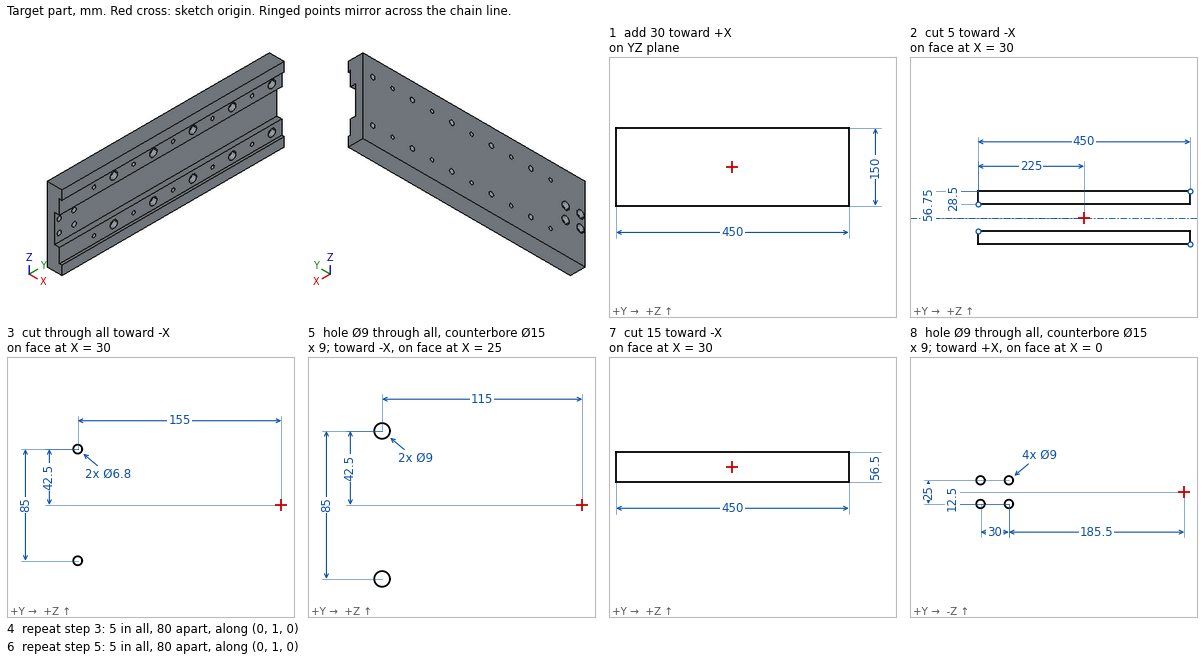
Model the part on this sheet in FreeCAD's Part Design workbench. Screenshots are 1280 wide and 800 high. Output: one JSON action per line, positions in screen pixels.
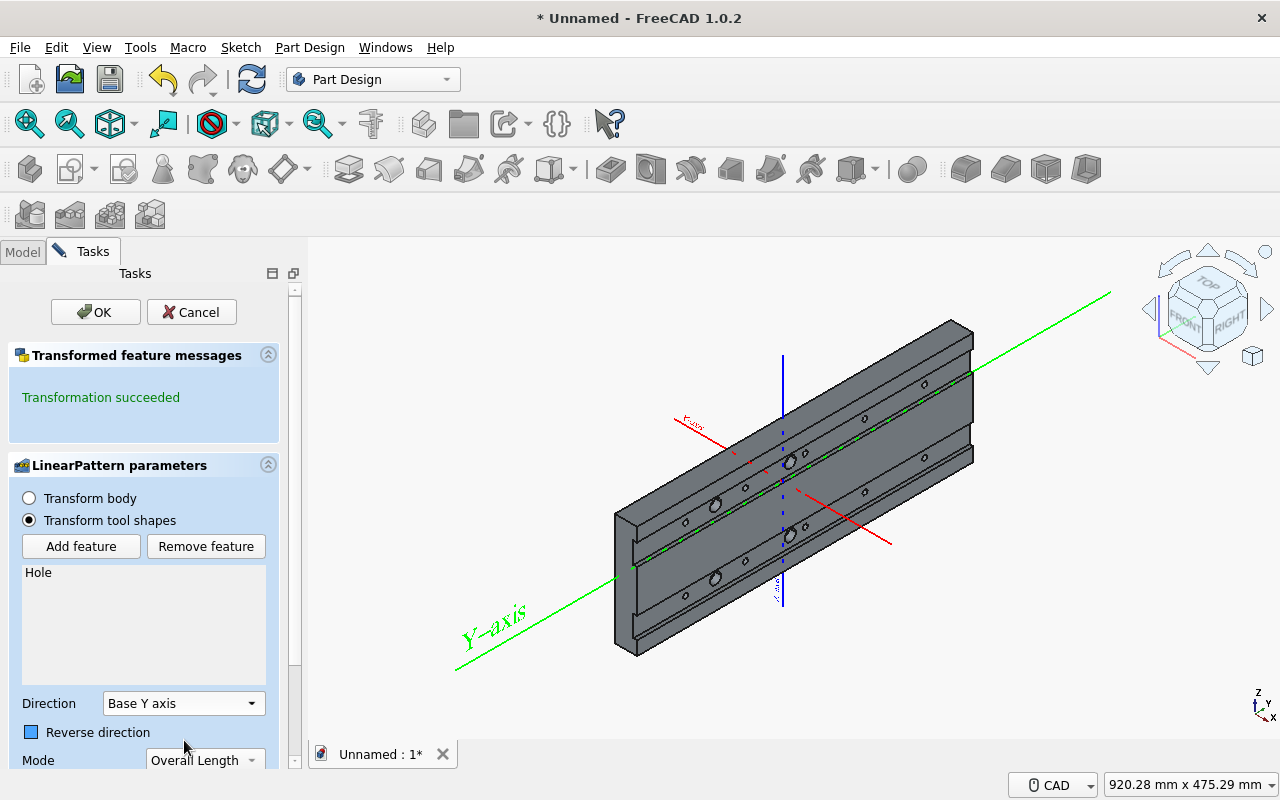
{"action": "scroll", "coordinate": [295, 526], "scroll_direction": "down", "scroll_amount": 2}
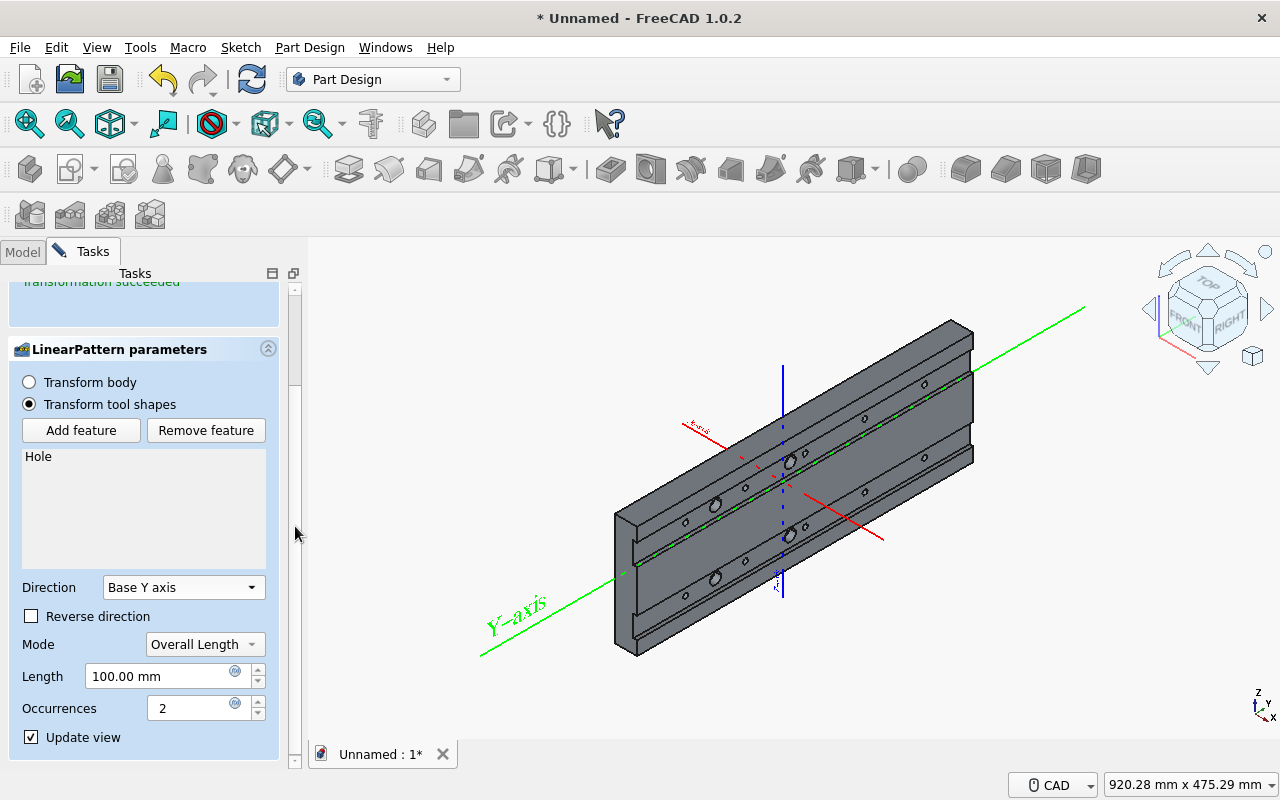
{"action": "left_click", "coordinate": [206, 644]}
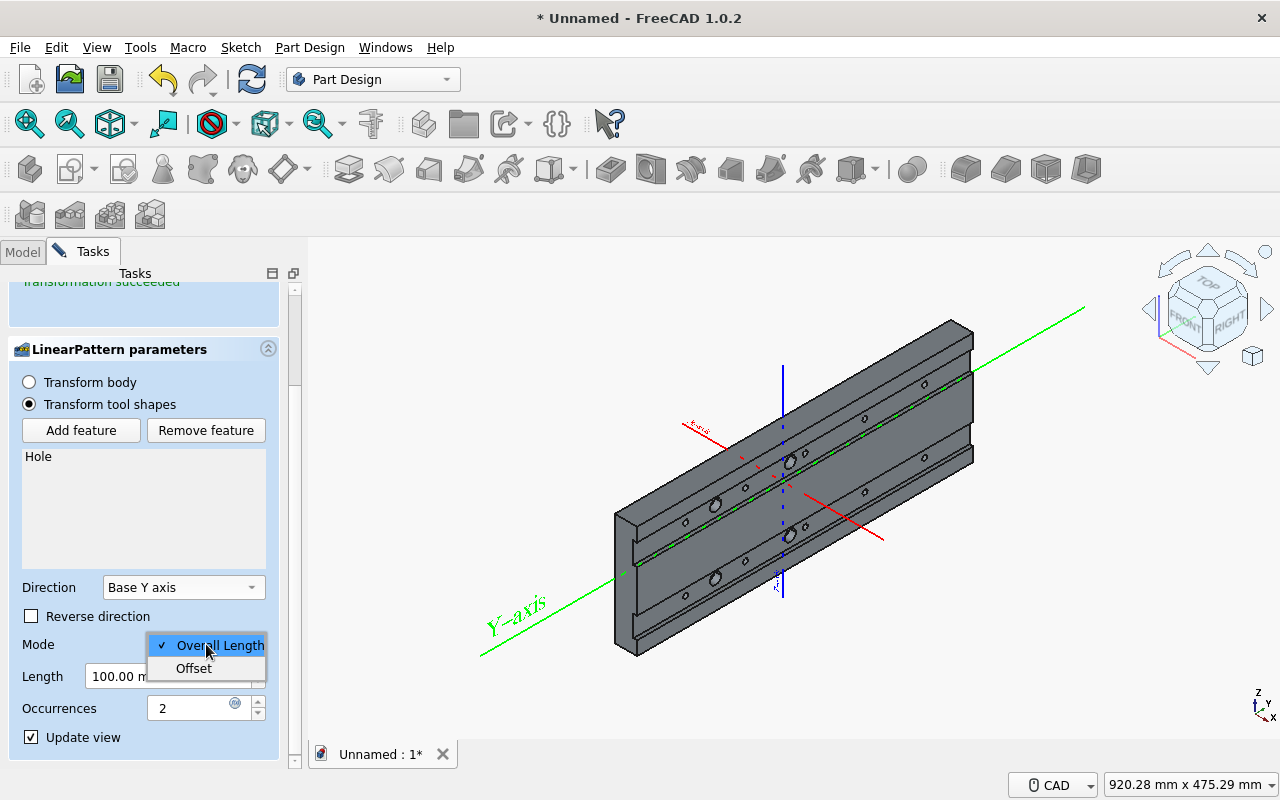
{"action": "left_click", "coordinate": [206, 668]}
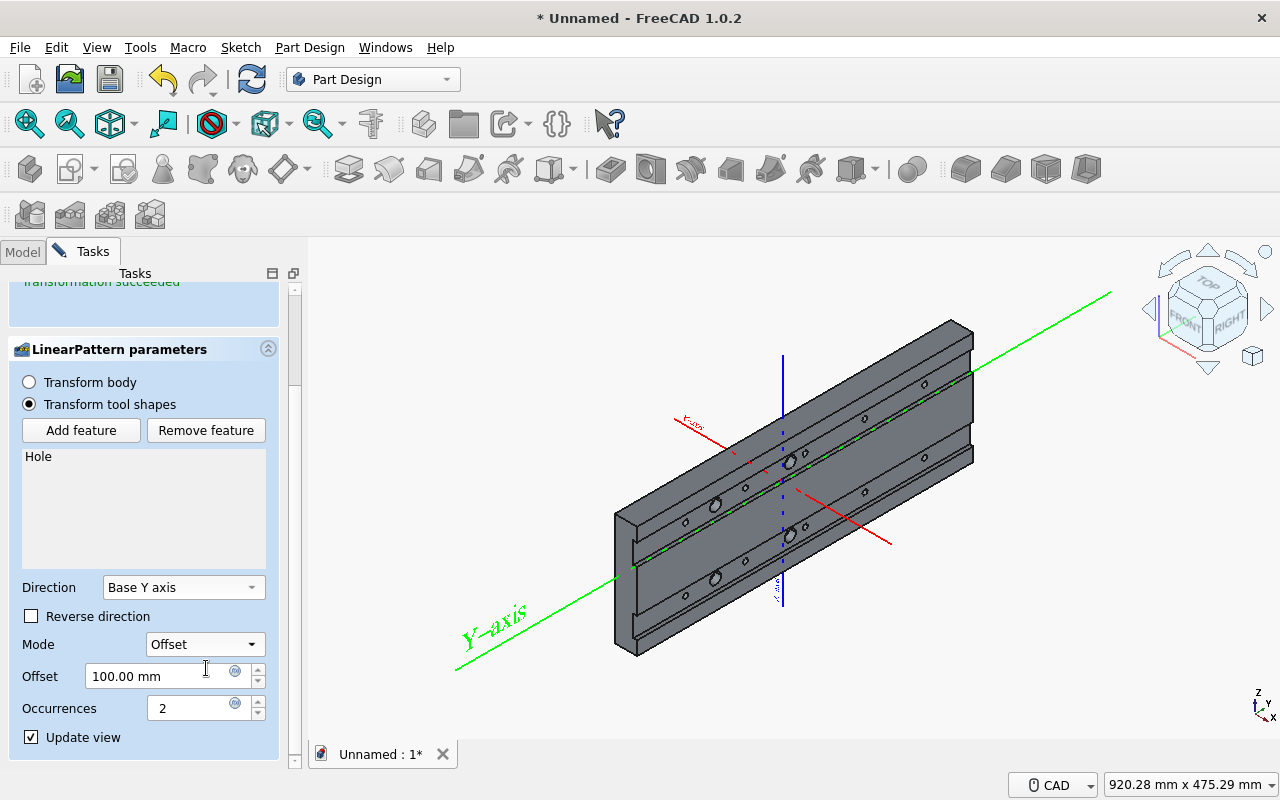
{"action": "triple_click", "coordinate": [168, 676]}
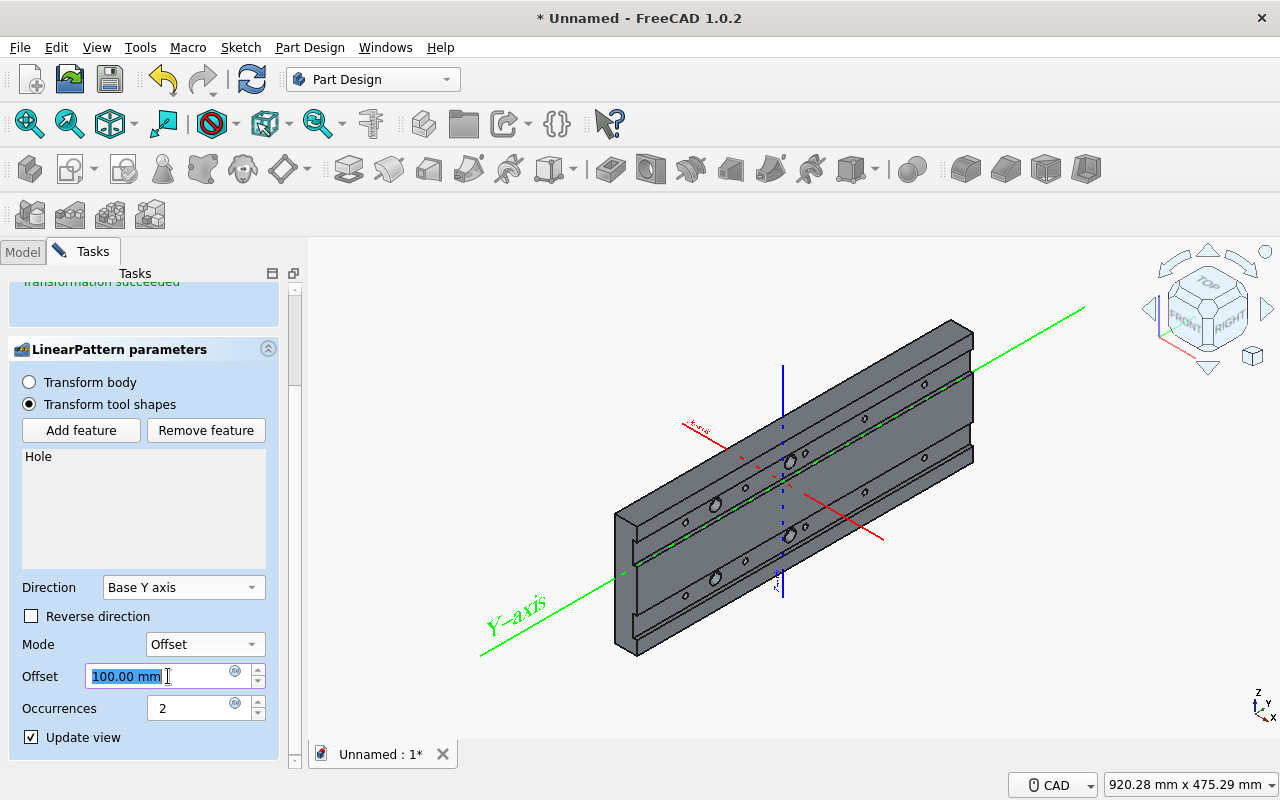
{"action": "type", "text": "80"}
{"action": "key", "text": "Tab"}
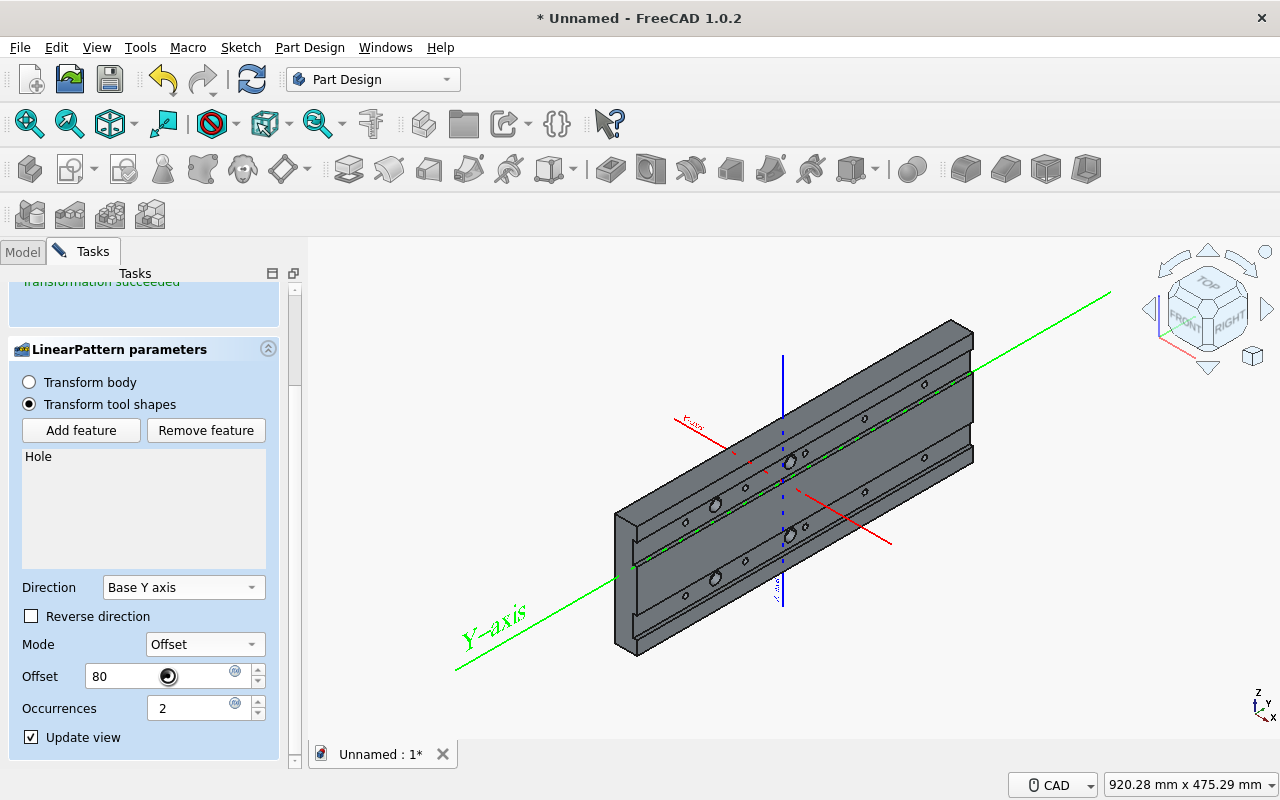
{"action": "triple_click", "coordinate": [198, 708]}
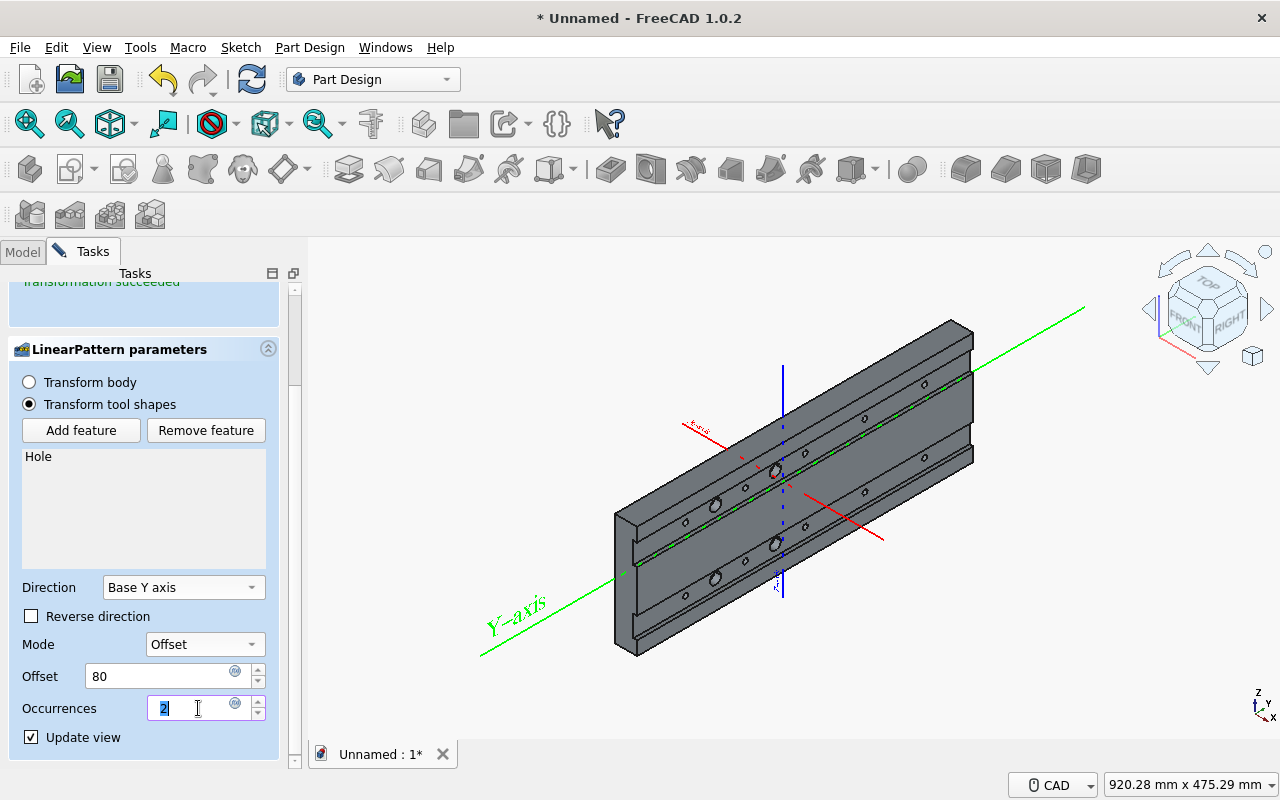
{"action": "type", "text": "5"}
{"action": "key", "text": "Tab"}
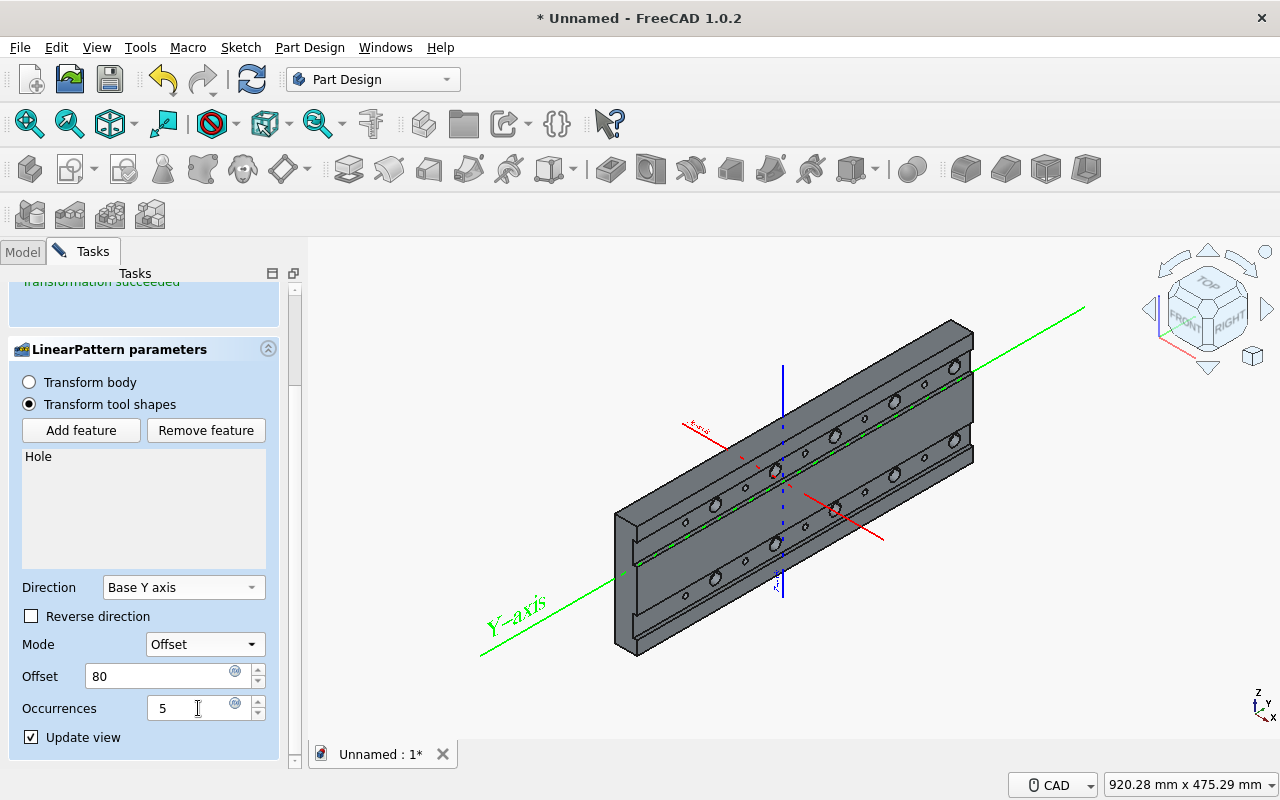
{"action": "scroll", "coordinate": [295, 526], "scroll_direction": "up", "scroll_amount": 3}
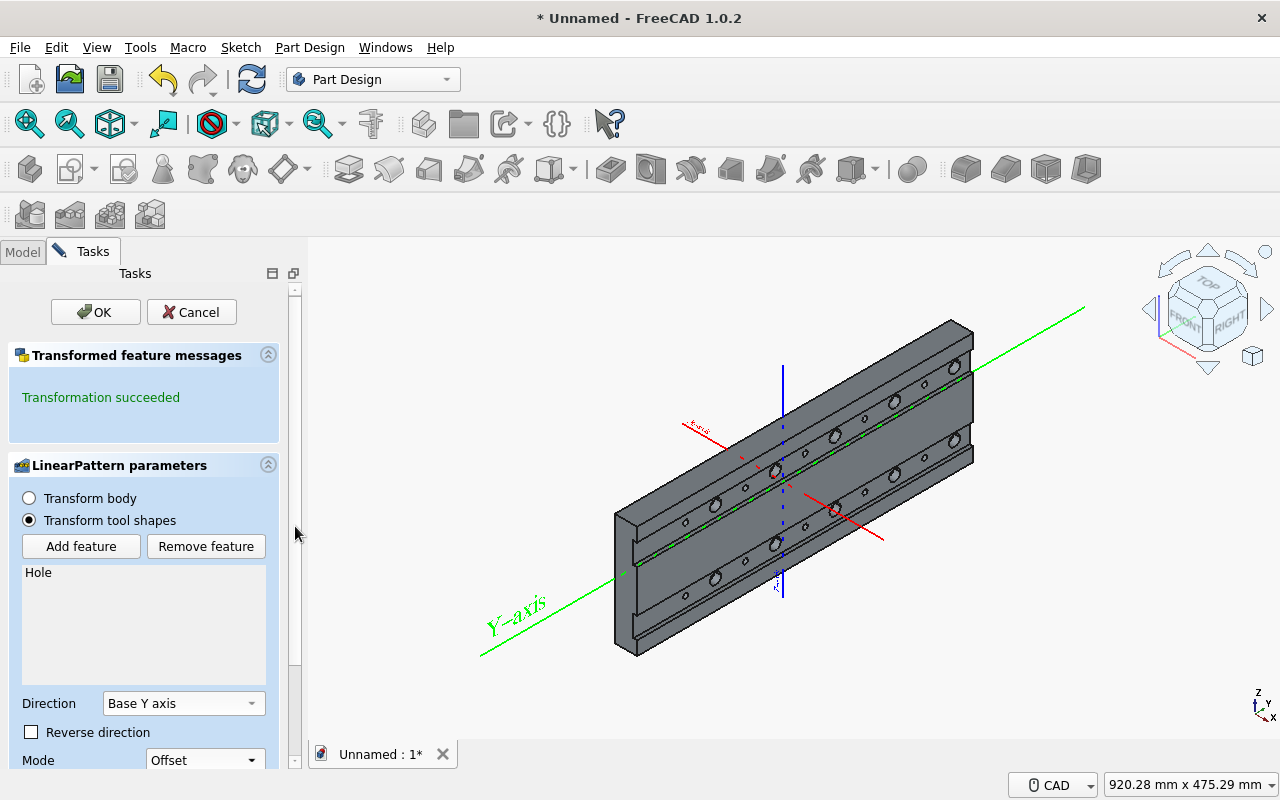
{"action": "left_click", "coordinate": [96, 312]}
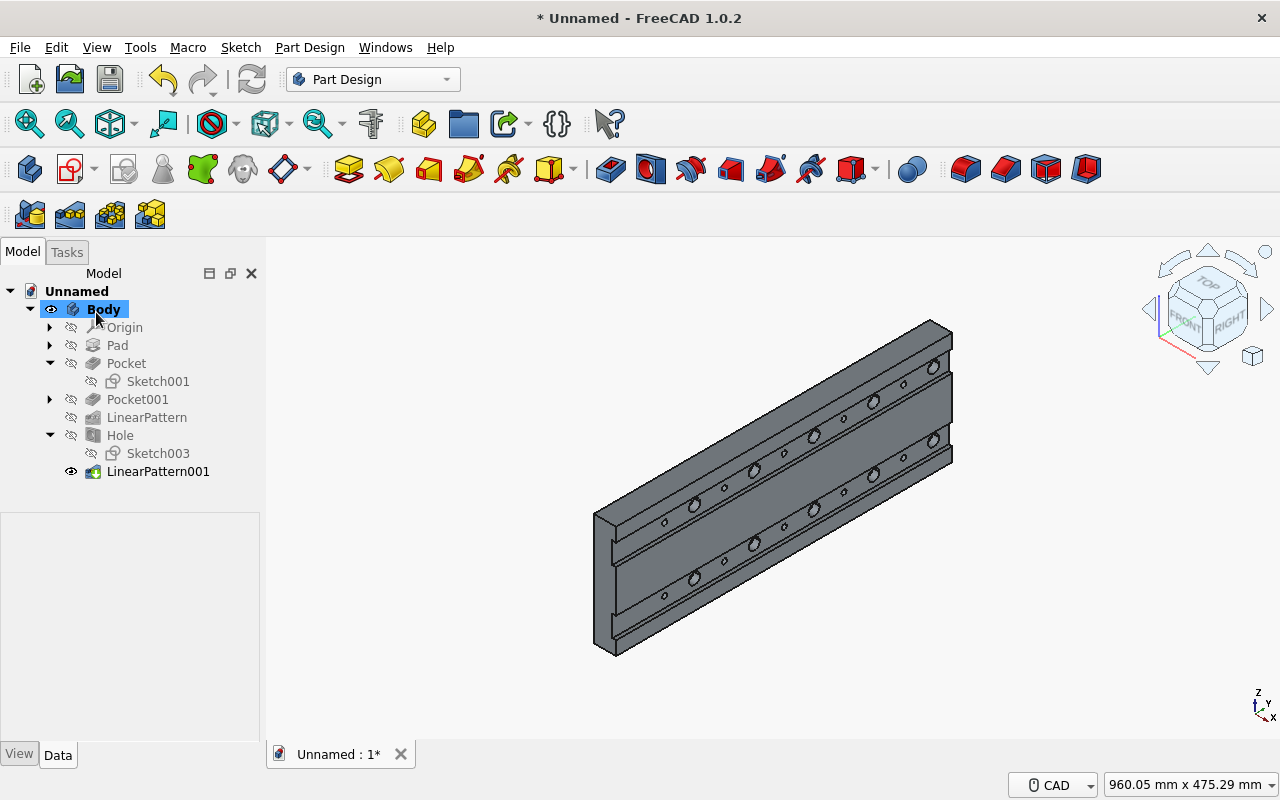
{"action": "left_click", "coordinate": [784, 493]}